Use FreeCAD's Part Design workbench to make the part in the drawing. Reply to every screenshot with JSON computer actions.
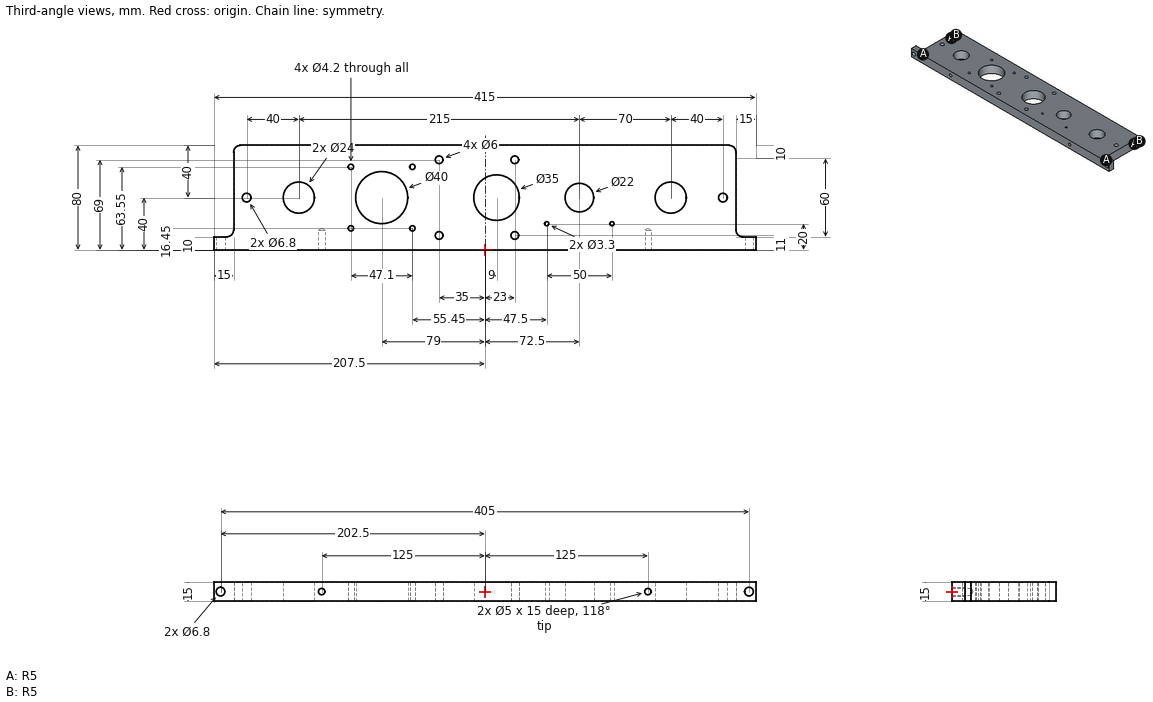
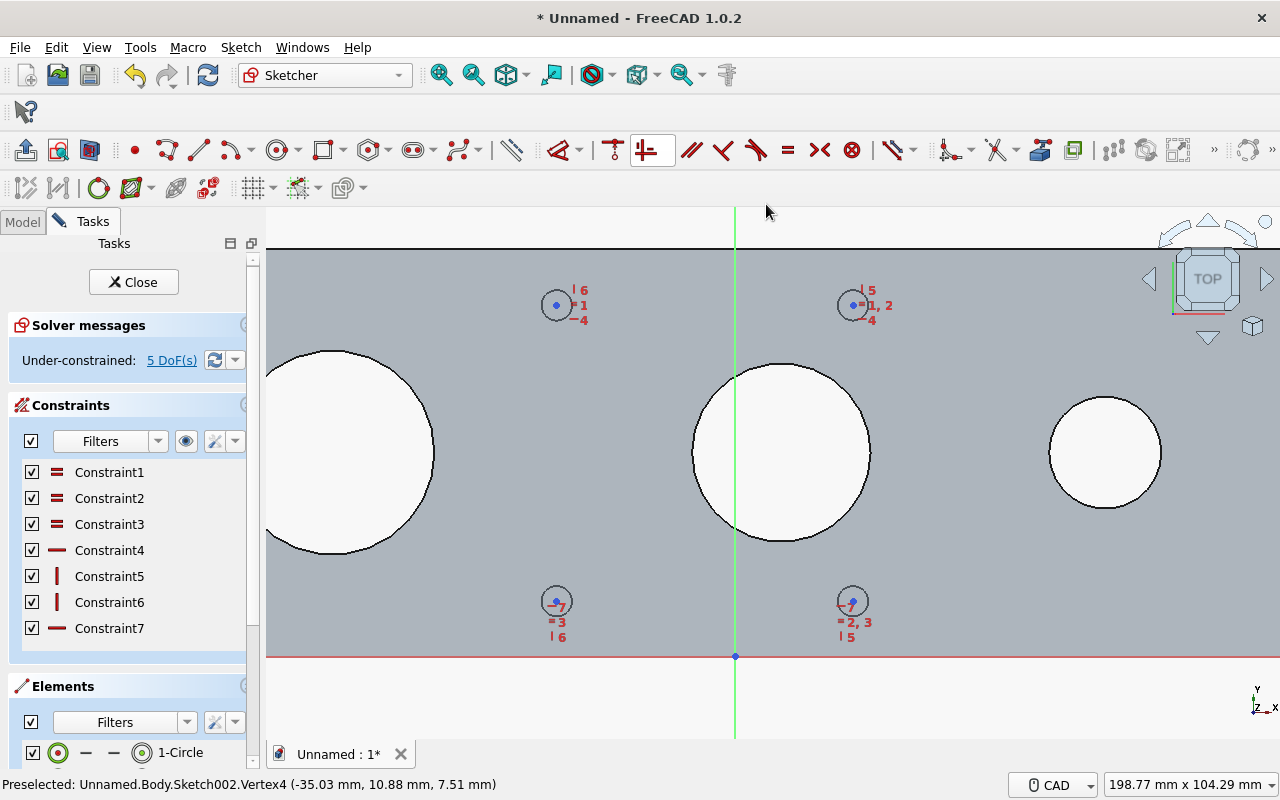
{"action": "left_click", "coordinate": [558, 150]}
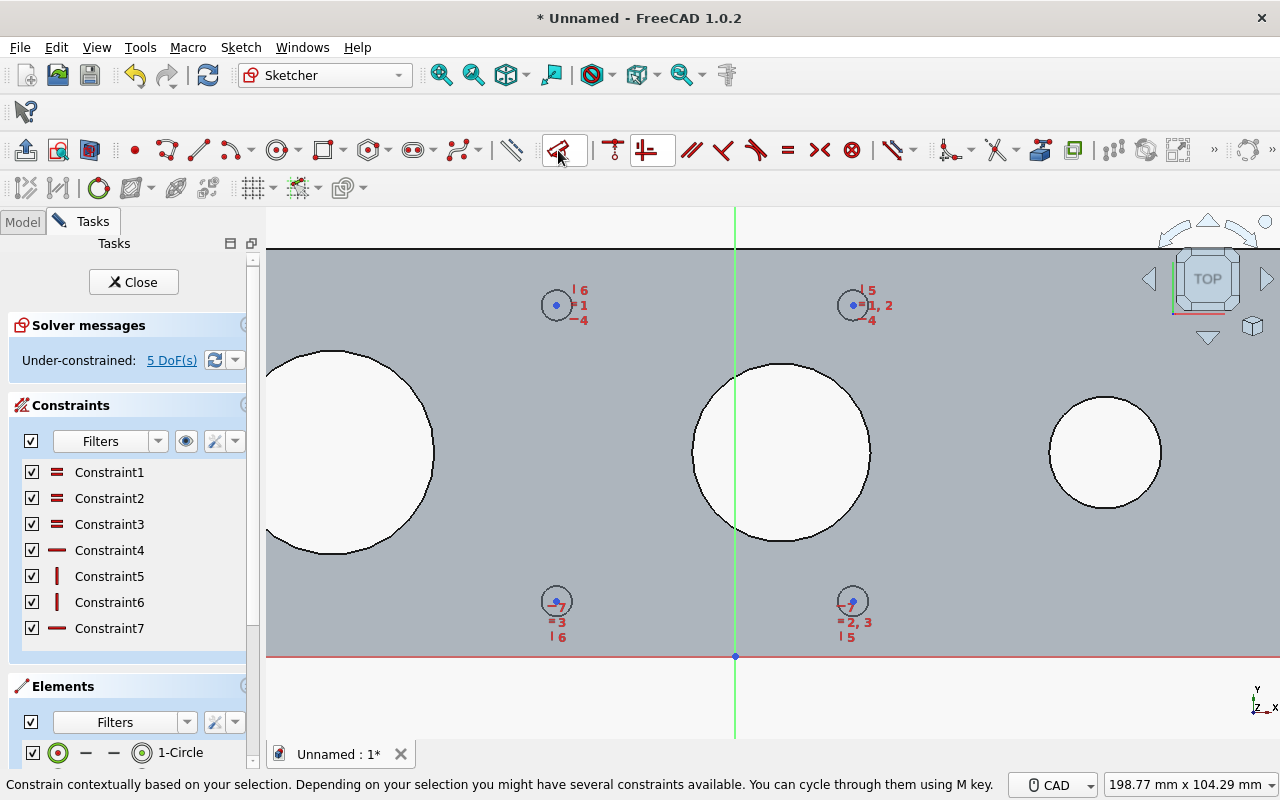
{"action": "scroll", "coordinate": [567, 295], "scroll_direction": "up", "scroll_amount": 2}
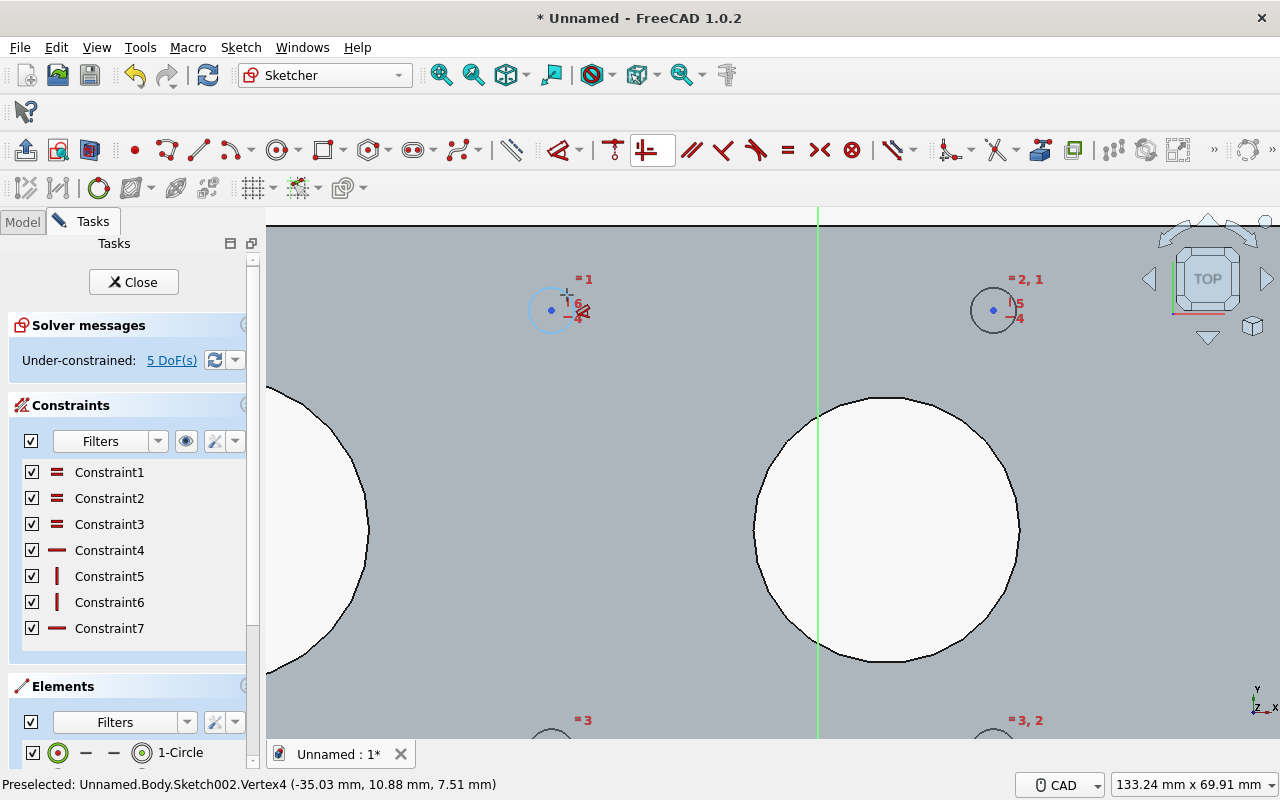
{"action": "left_click", "coordinate": [568, 294]}
{"action": "left_click", "coordinate": [591, 271]}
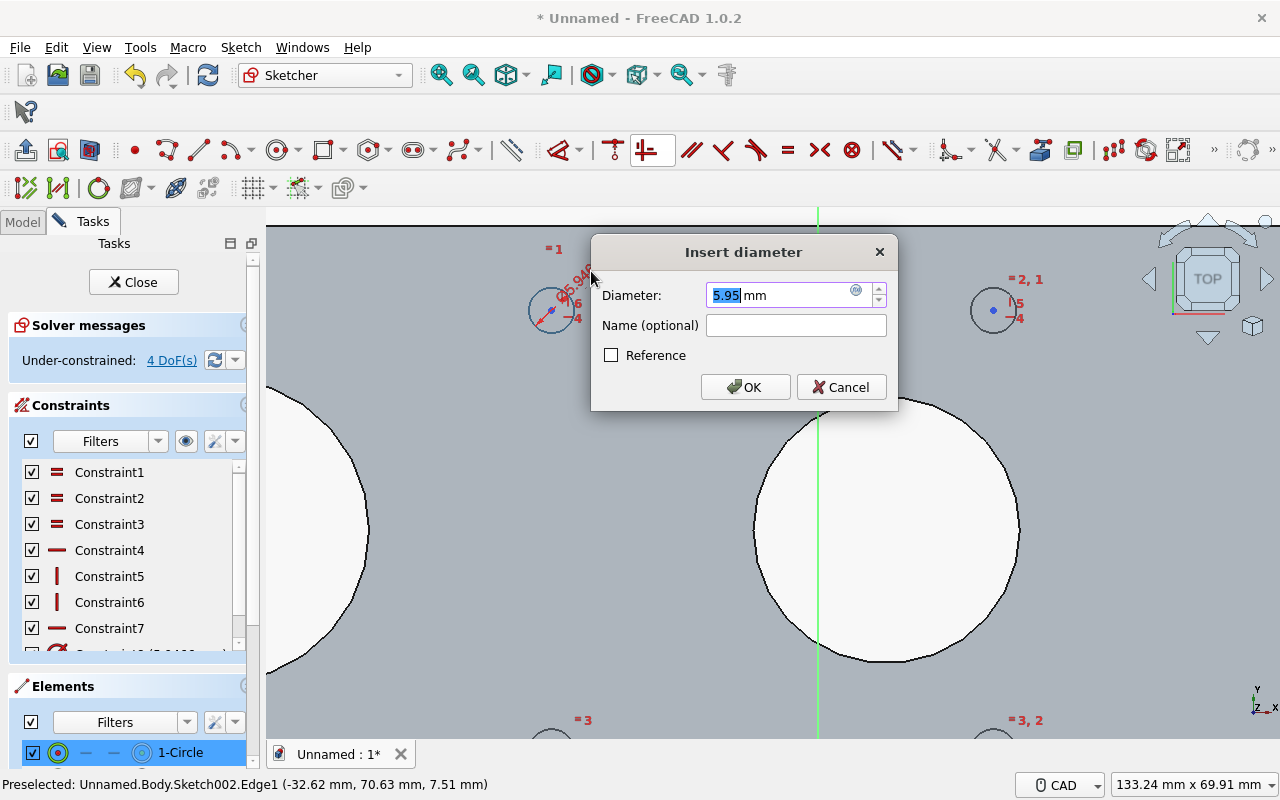
{"action": "type", "text": "6"}
{"action": "key", "text": "Return"}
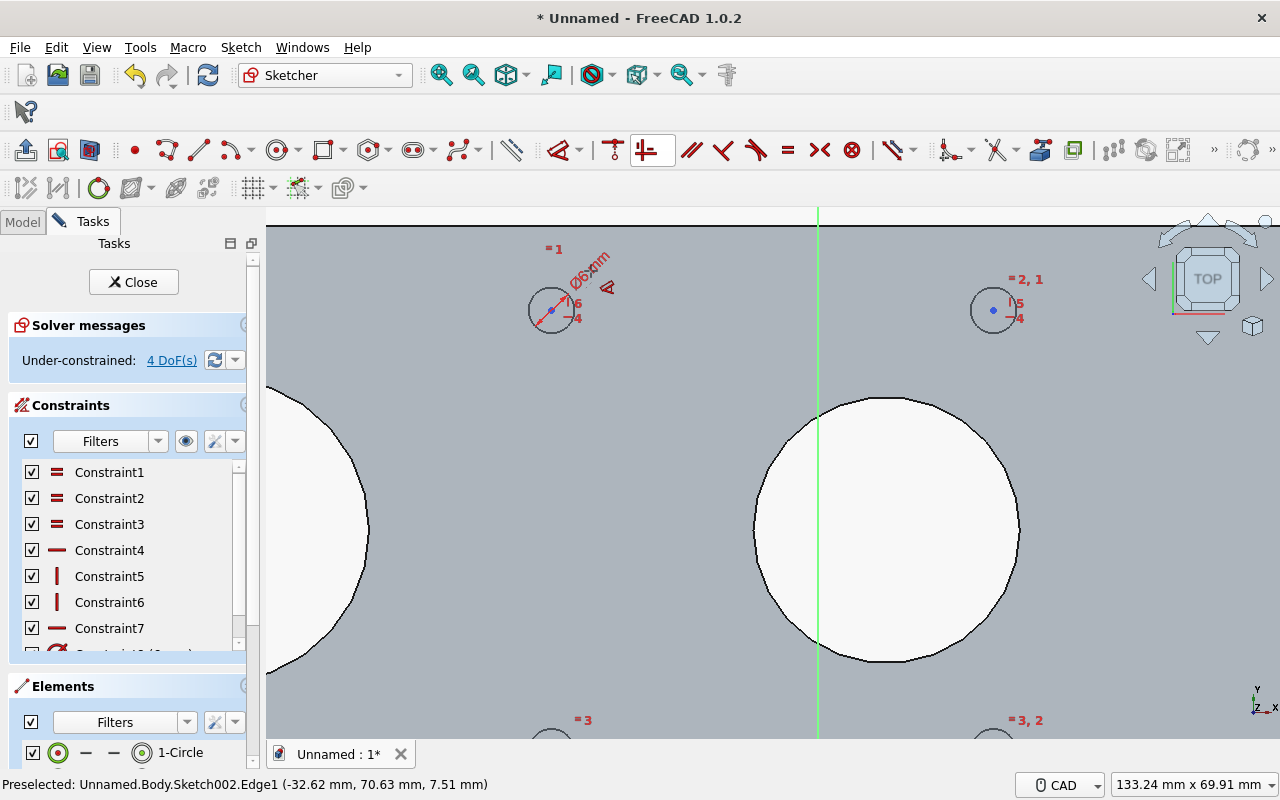
{"action": "left_click", "coordinate": [552, 310]}
{"action": "left_click", "coordinate": [685, 276]}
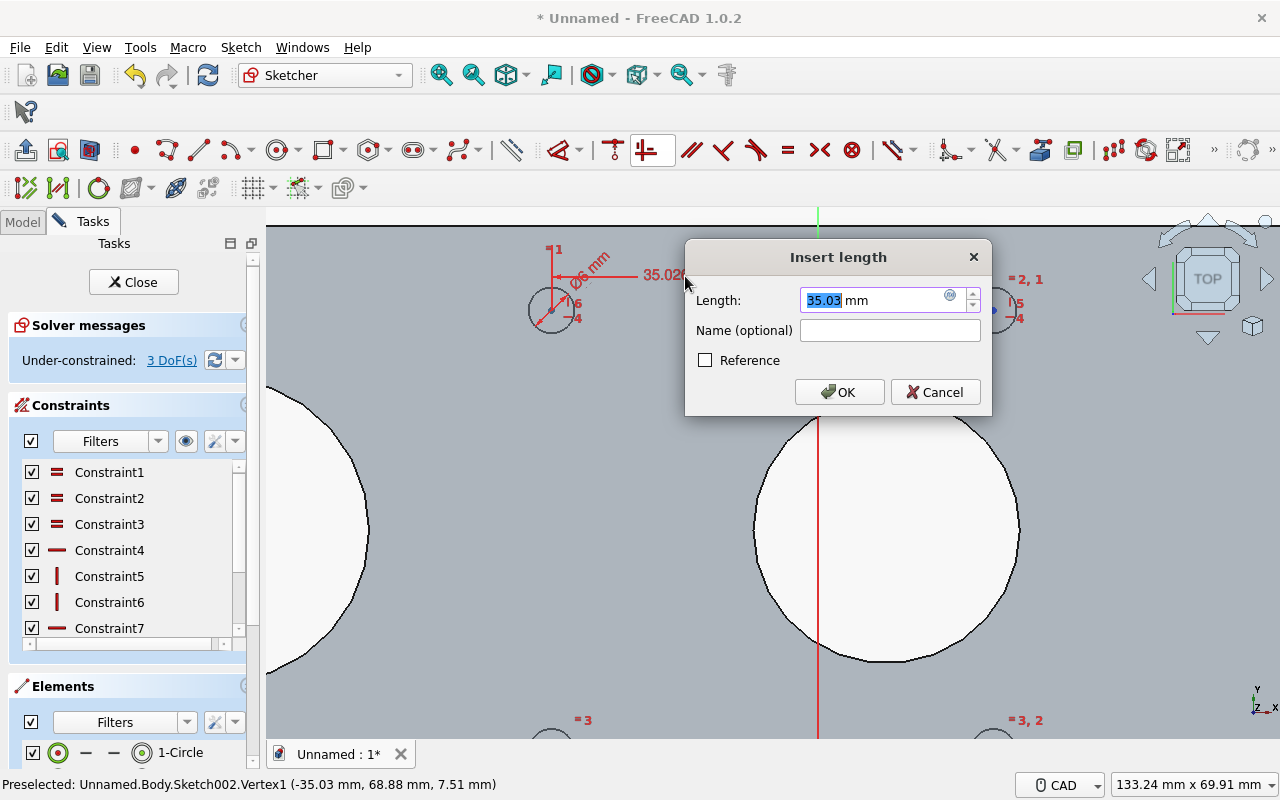
{"action": "type", "text": "35"}
{"action": "key", "text": "Return"}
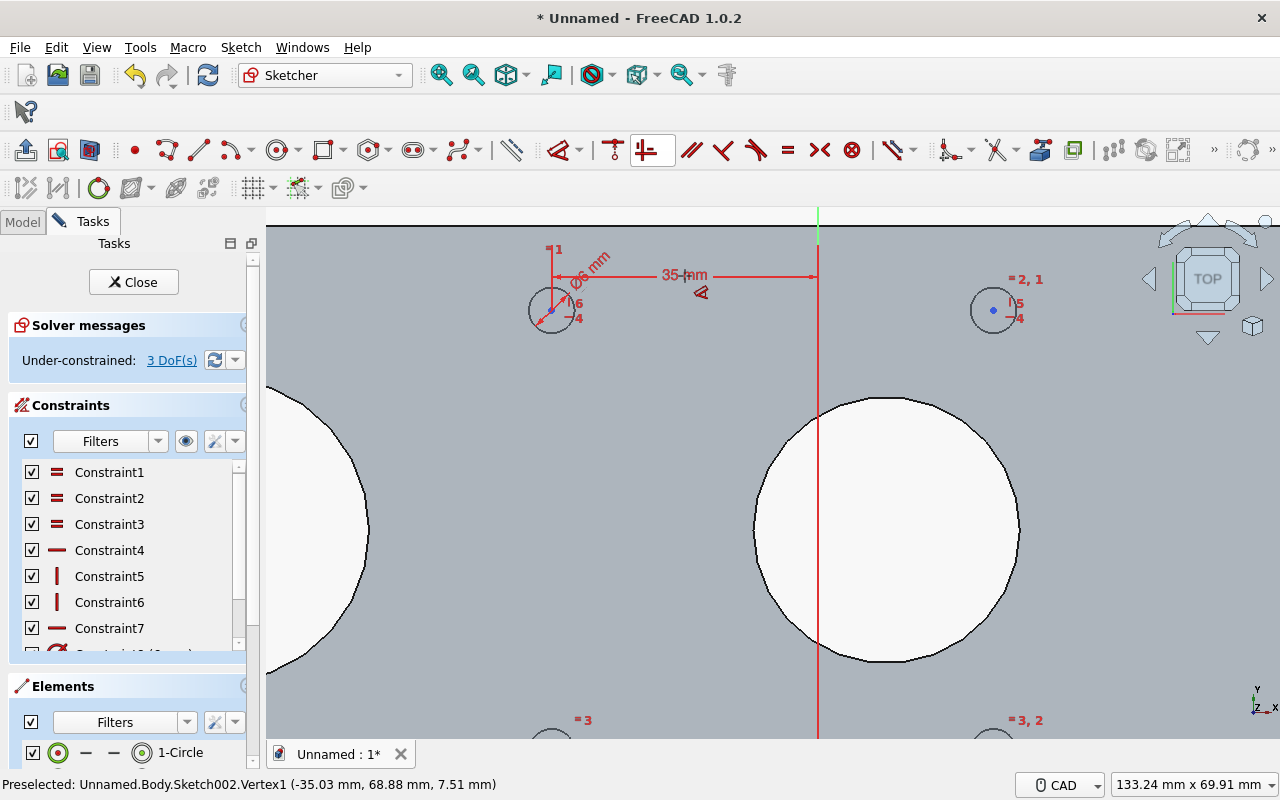
{"action": "left_click", "coordinate": [552, 310]}
{"action": "left_click", "coordinate": [518, 511]}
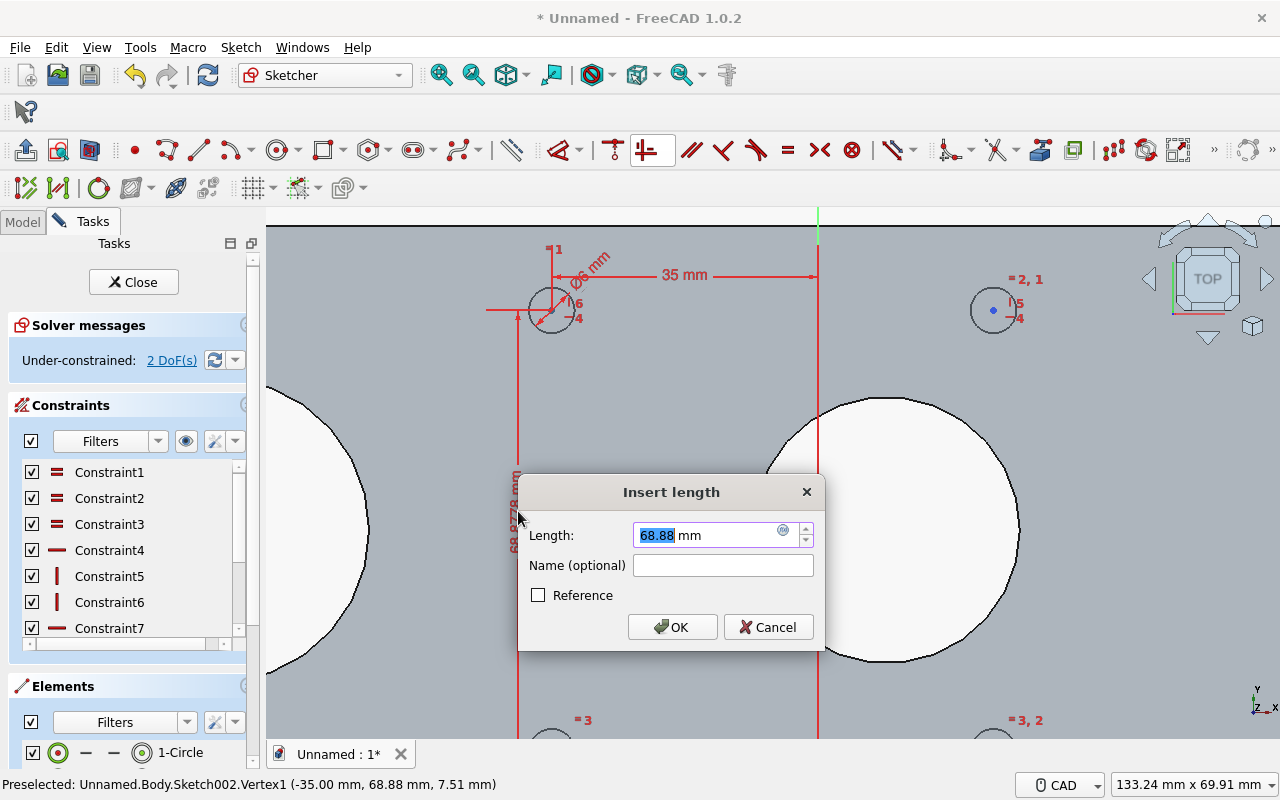
{"action": "type", "text": "69"}
{"action": "key", "text": "Return"}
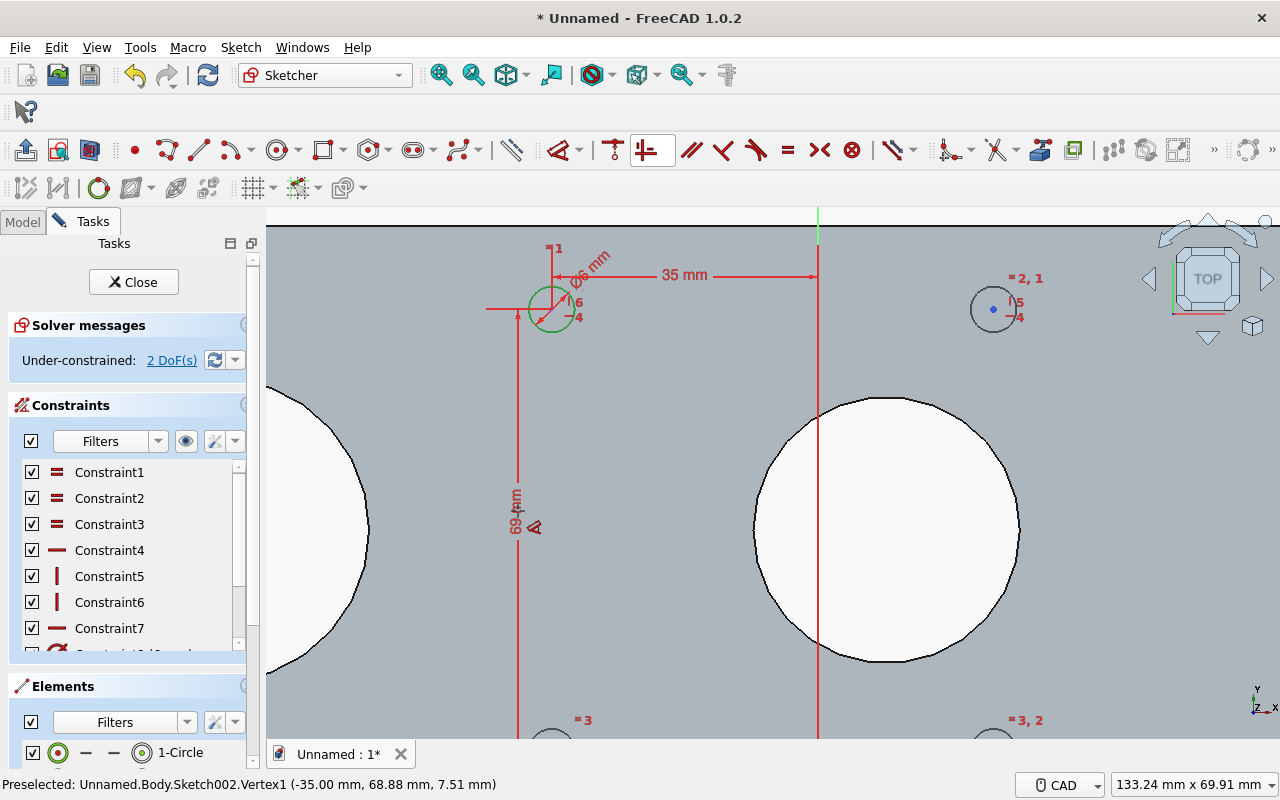
{"action": "left_click", "coordinate": [994, 309]}
{"action": "left_click", "coordinate": [906, 275]}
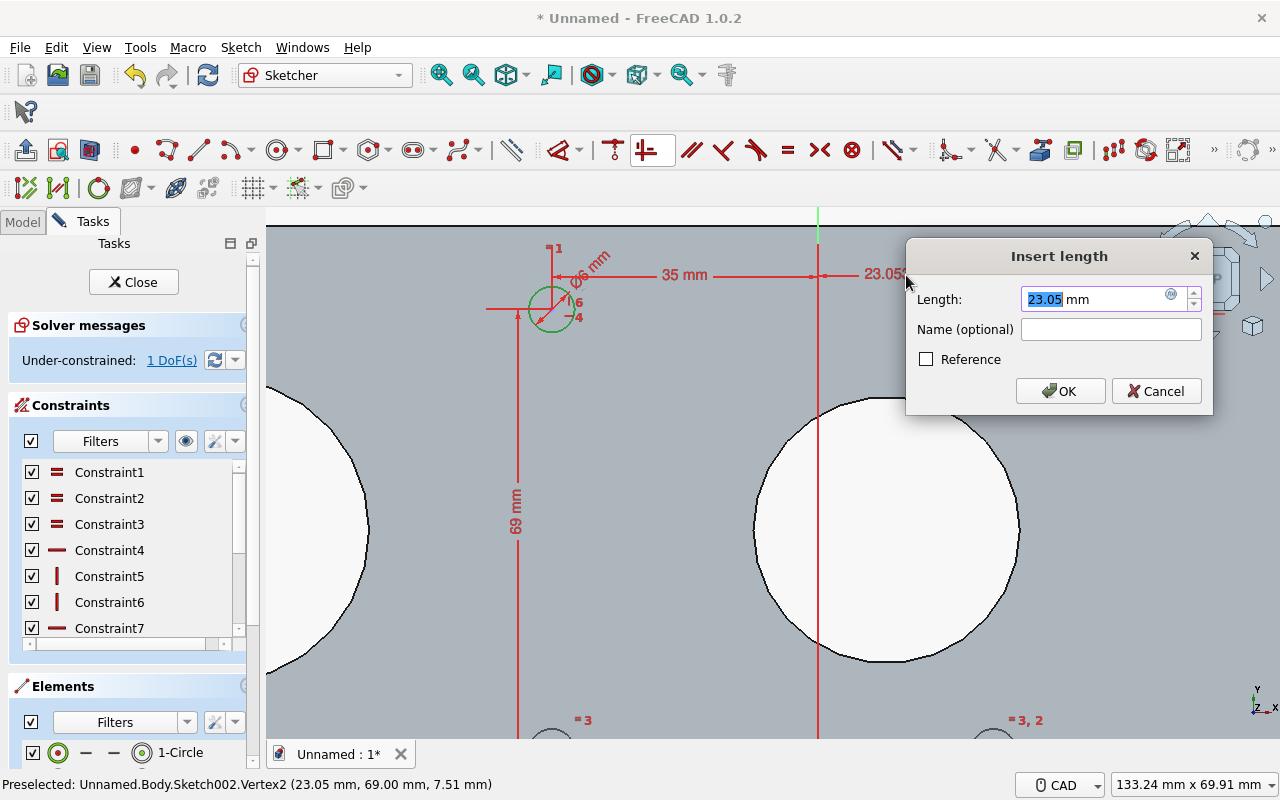
{"action": "type", "text": "23"}
{"action": "key", "text": "Return"}